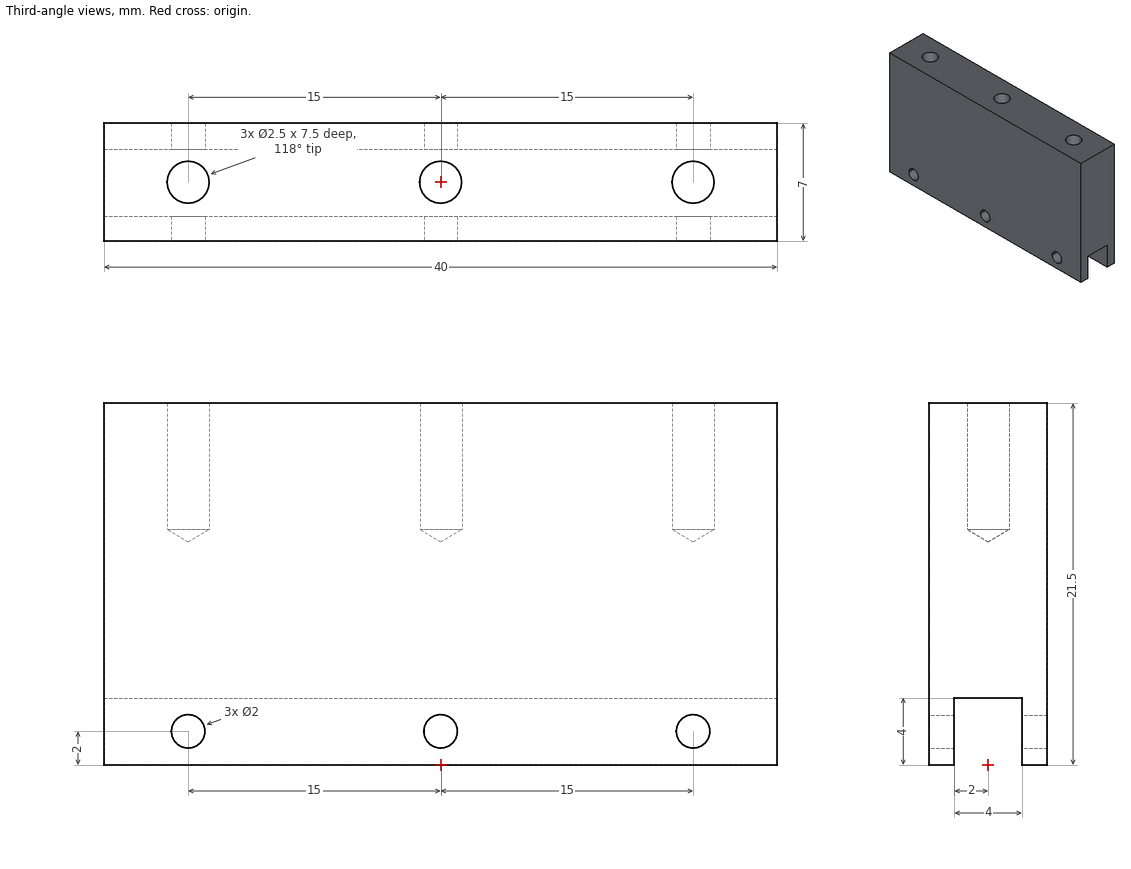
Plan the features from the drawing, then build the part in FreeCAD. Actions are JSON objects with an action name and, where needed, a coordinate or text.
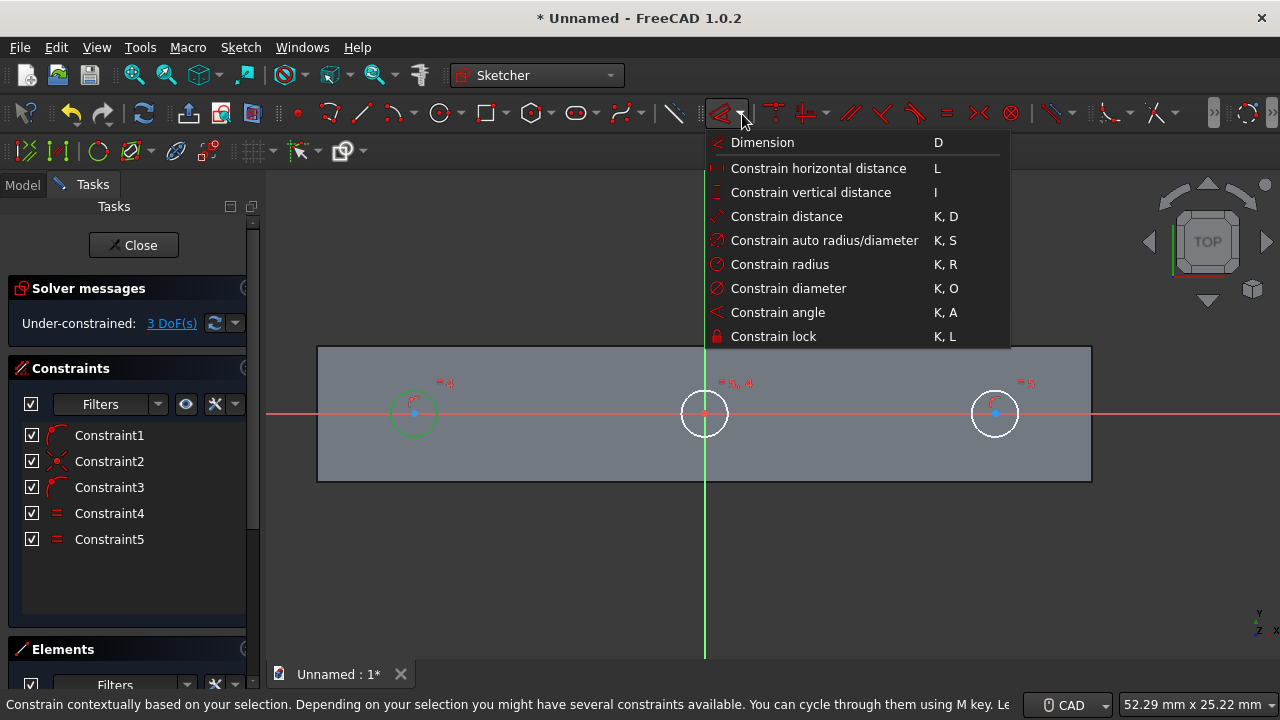
{"action": "left_click", "coordinate": [858, 288]}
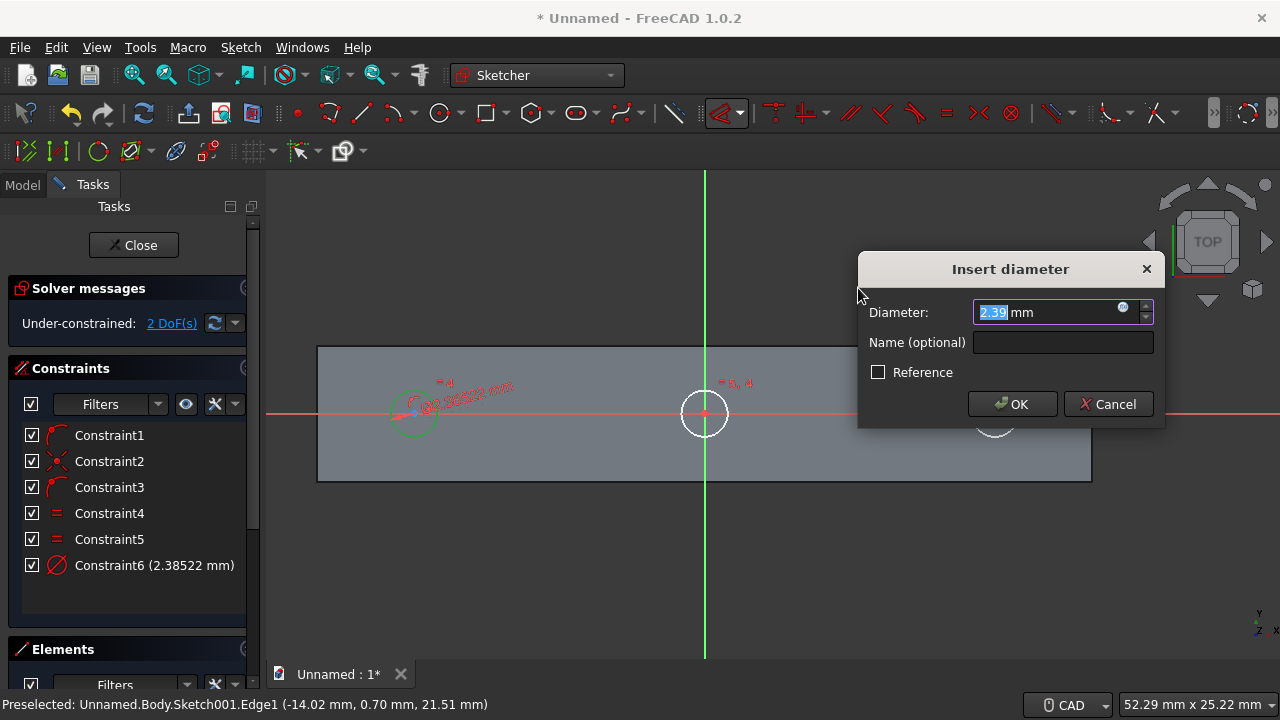
{"action": "type", "text": "2.5"}
{"action": "key", "text": "Return"}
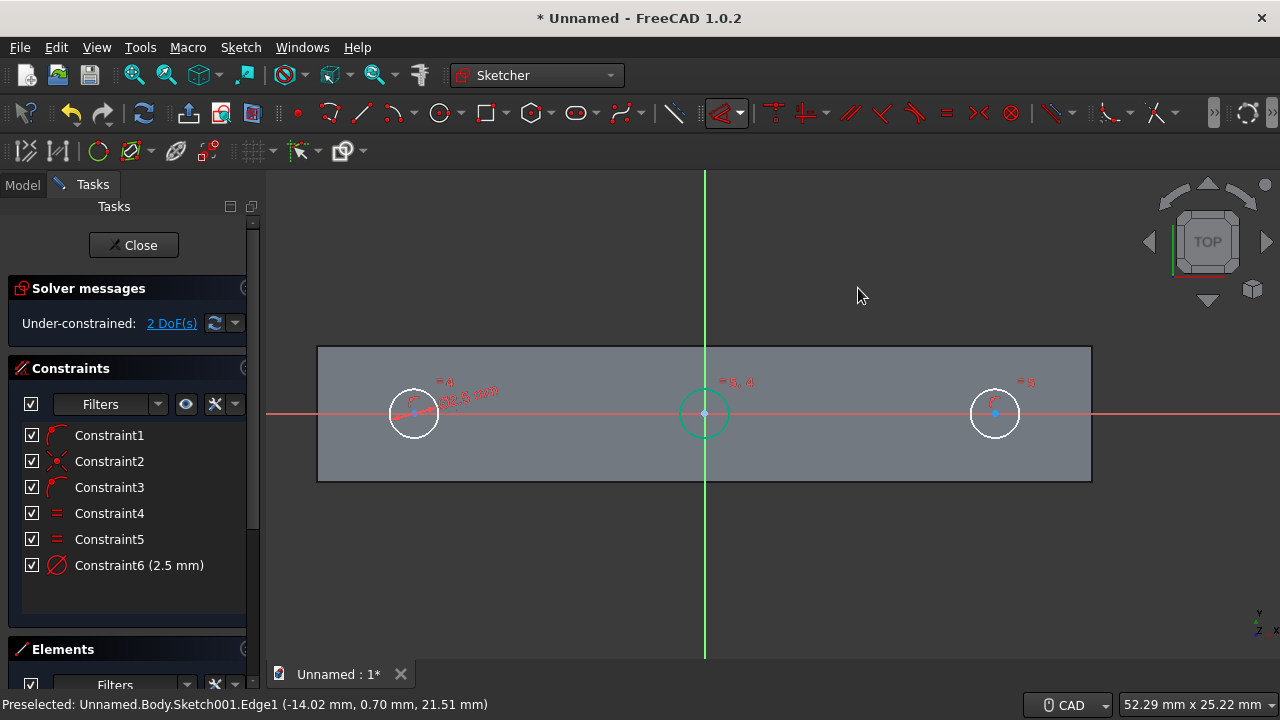
{"action": "left_click", "coordinate": [414, 414]}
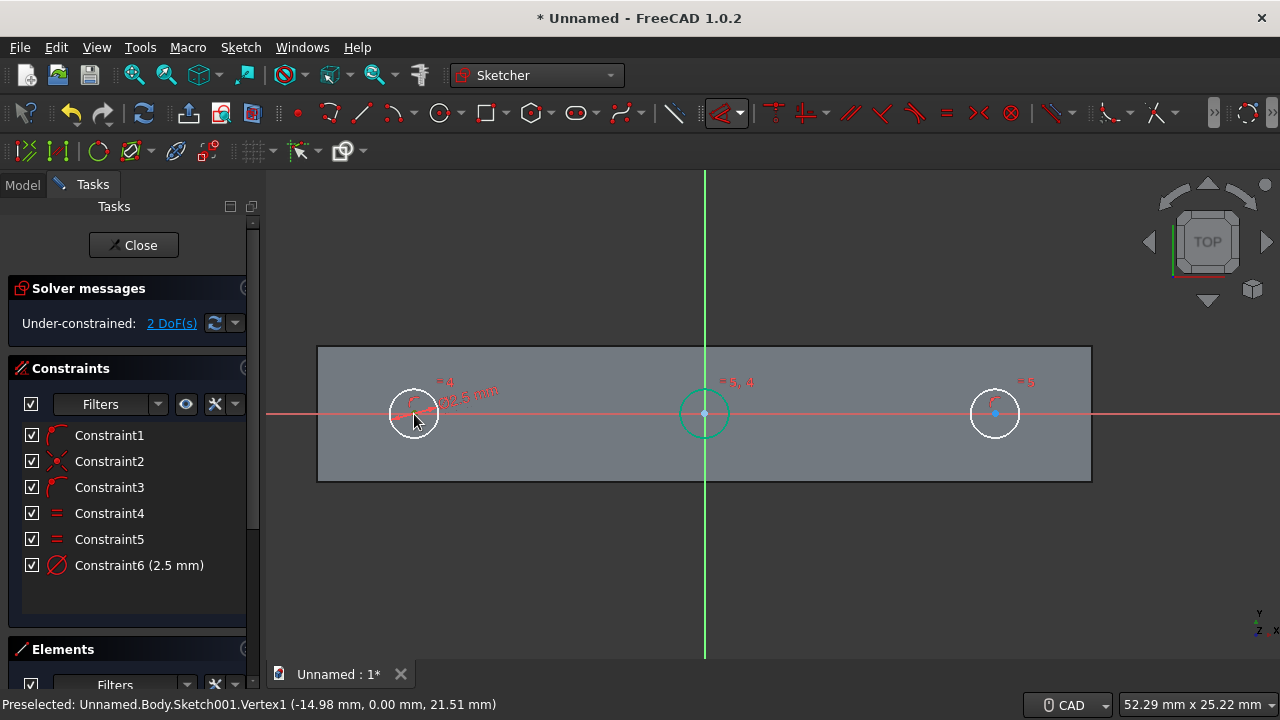
{"action": "left_click", "coordinate": [742, 114]}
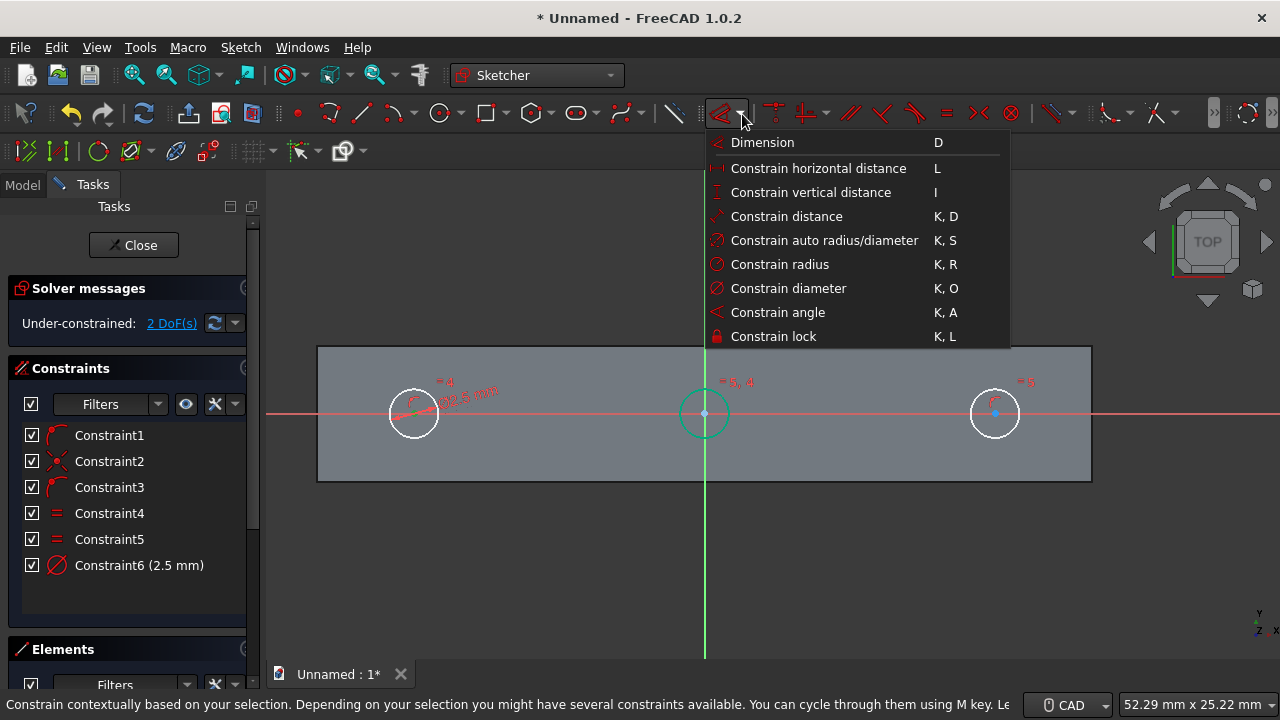
{"action": "left_click", "coordinate": [858, 168]}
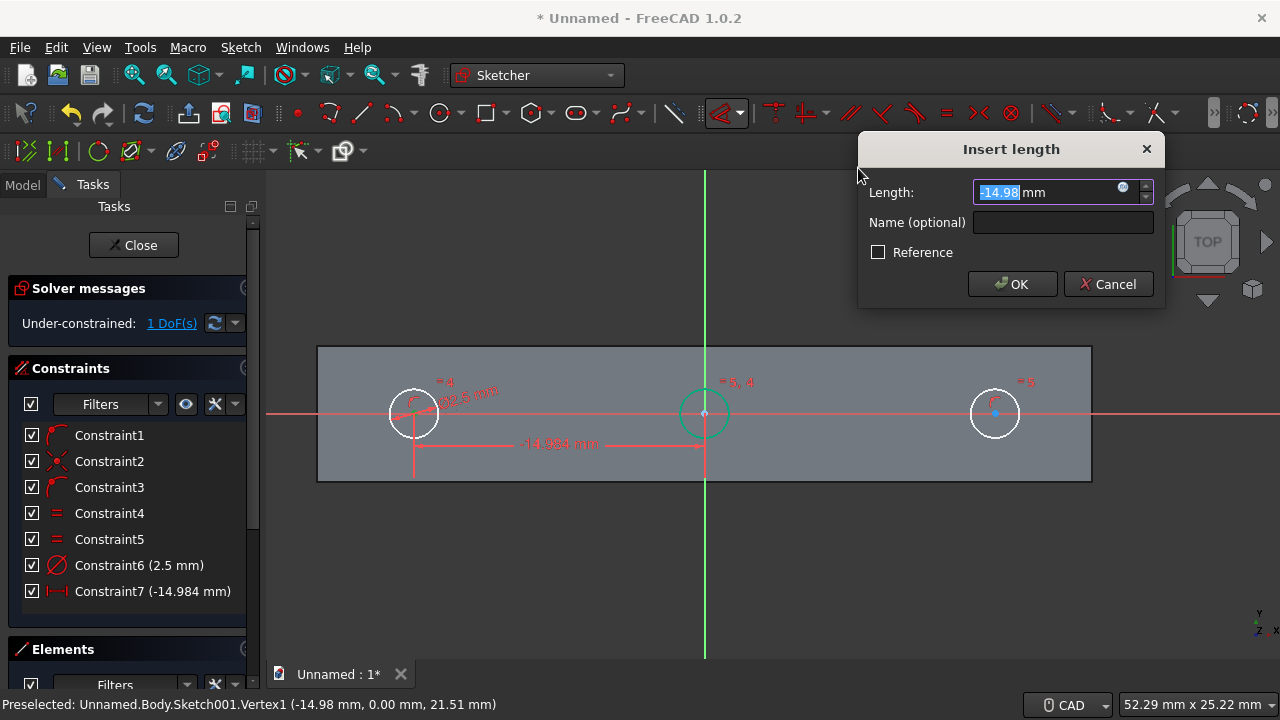
{"action": "type", "text": "-15"}
{"action": "key", "text": "Return"}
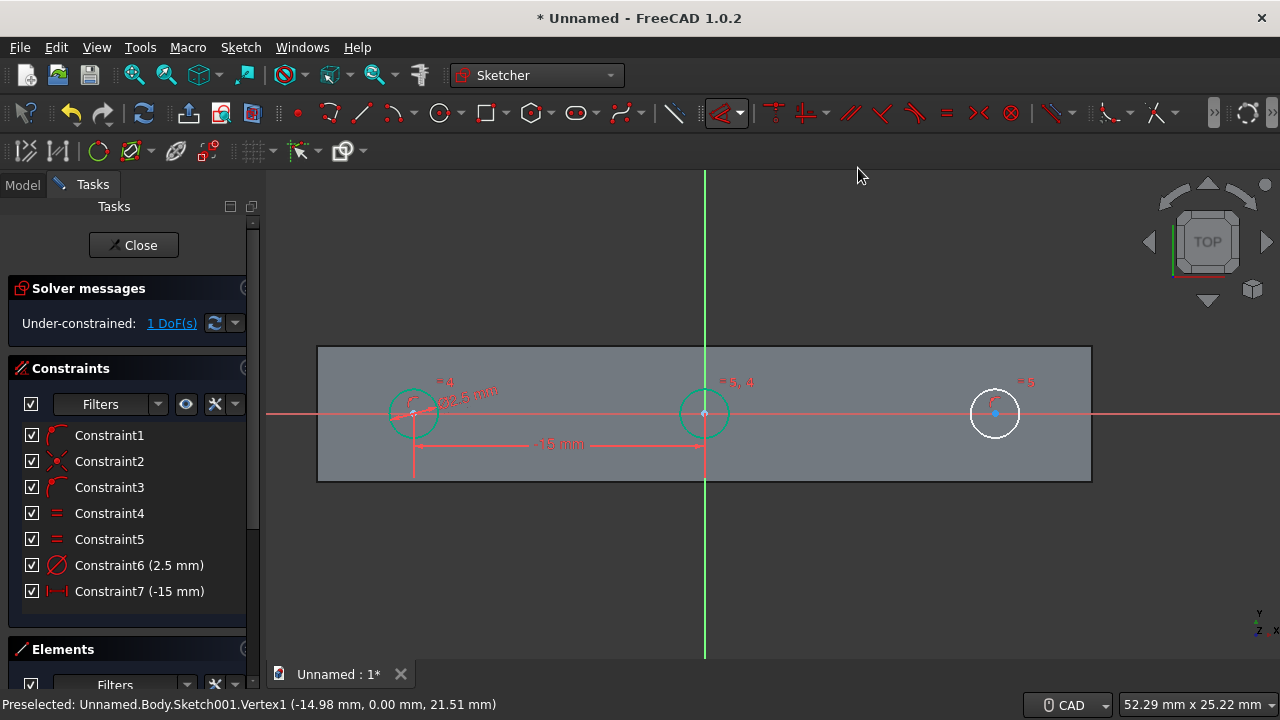
{"action": "left_click", "coordinate": [995, 414]}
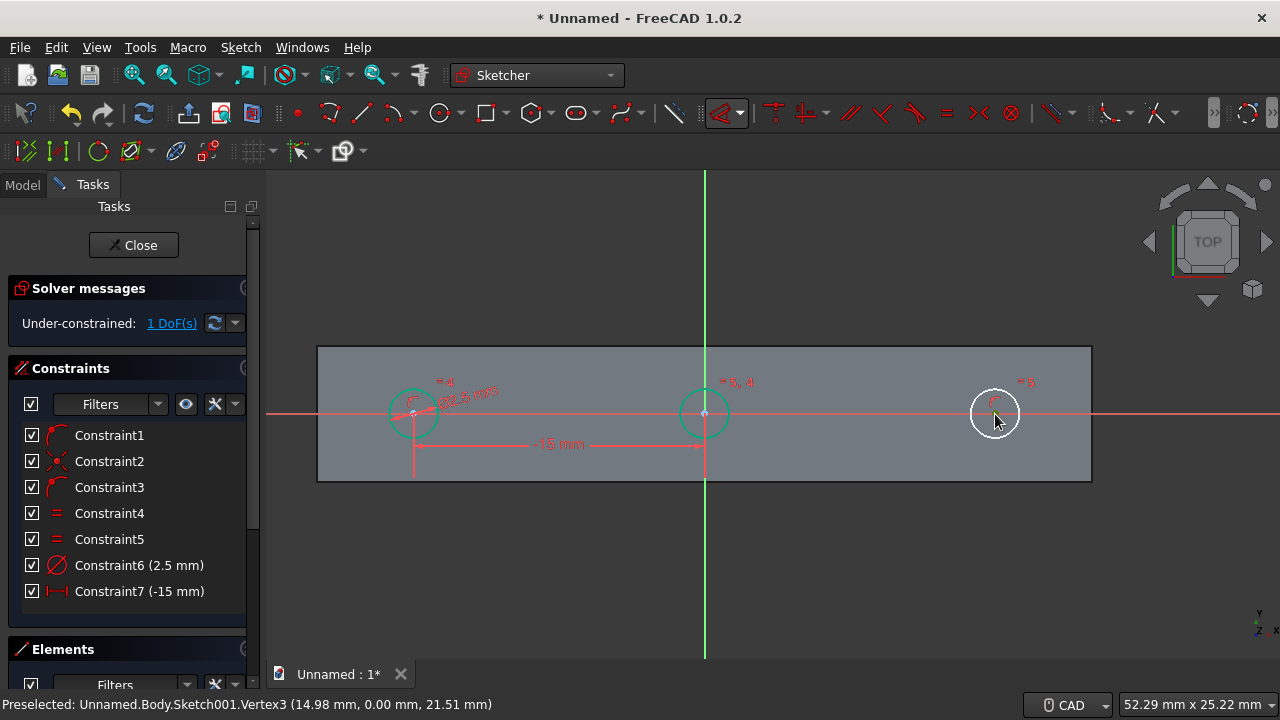
{"action": "left_click", "coordinate": [742, 114]}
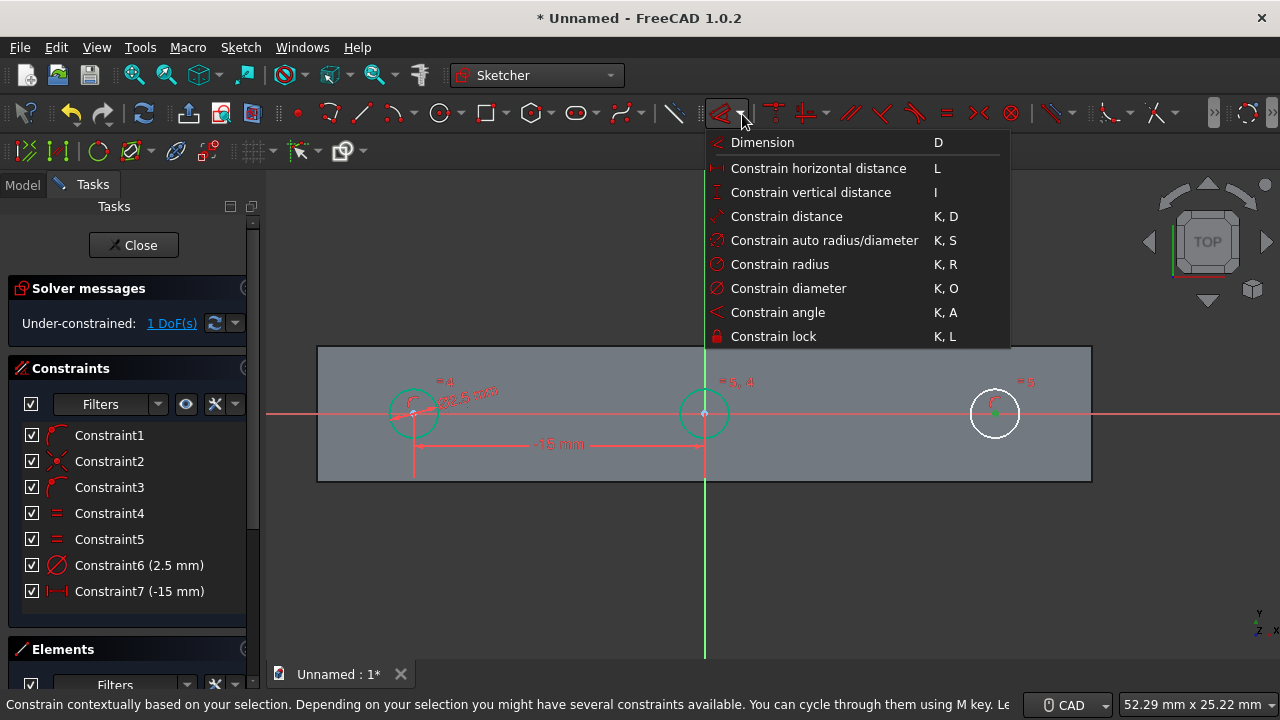
{"action": "left_click", "coordinate": [858, 168]}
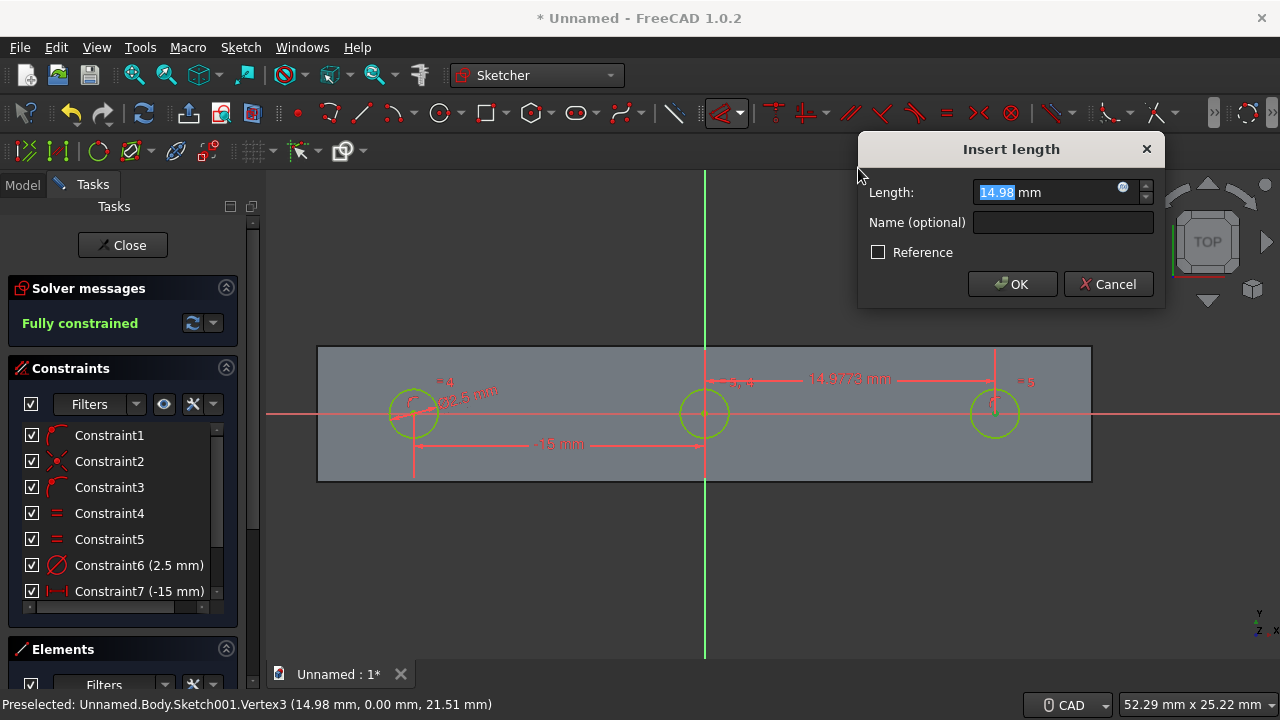
{"action": "type", "text": "15"}
{"action": "key", "text": "Return"}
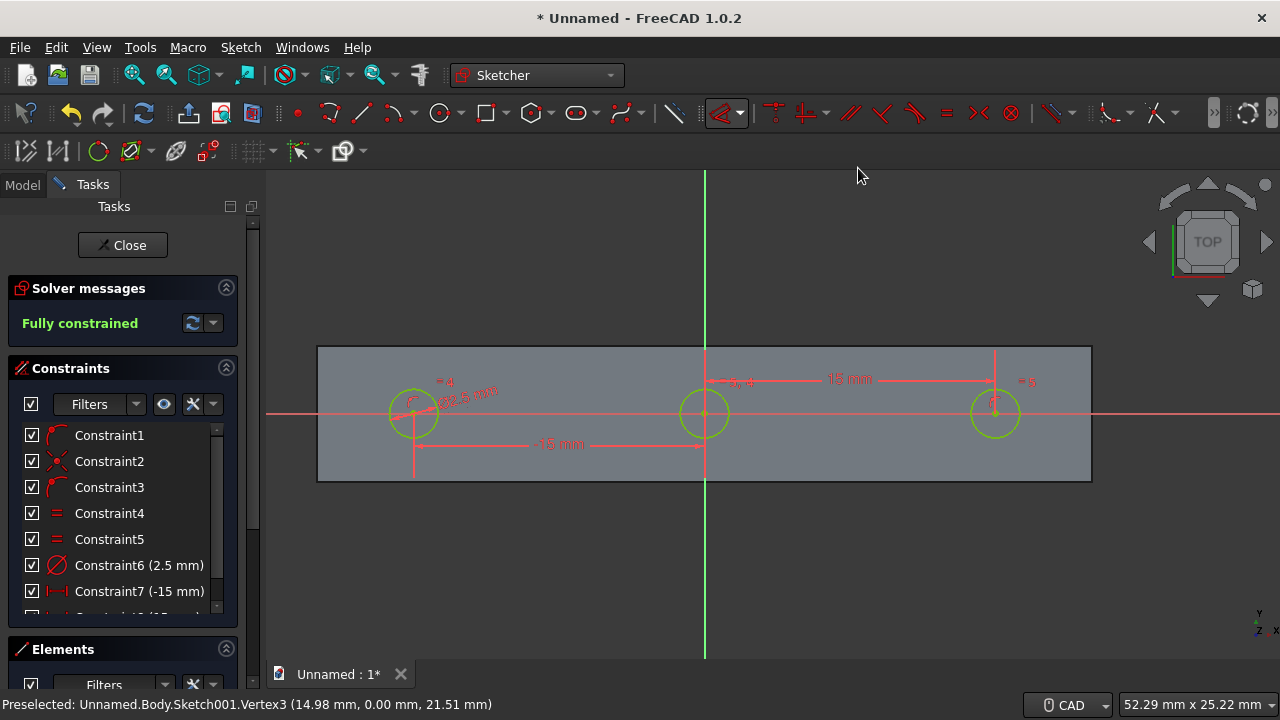
{"action": "left_click", "coordinate": [123, 245]}